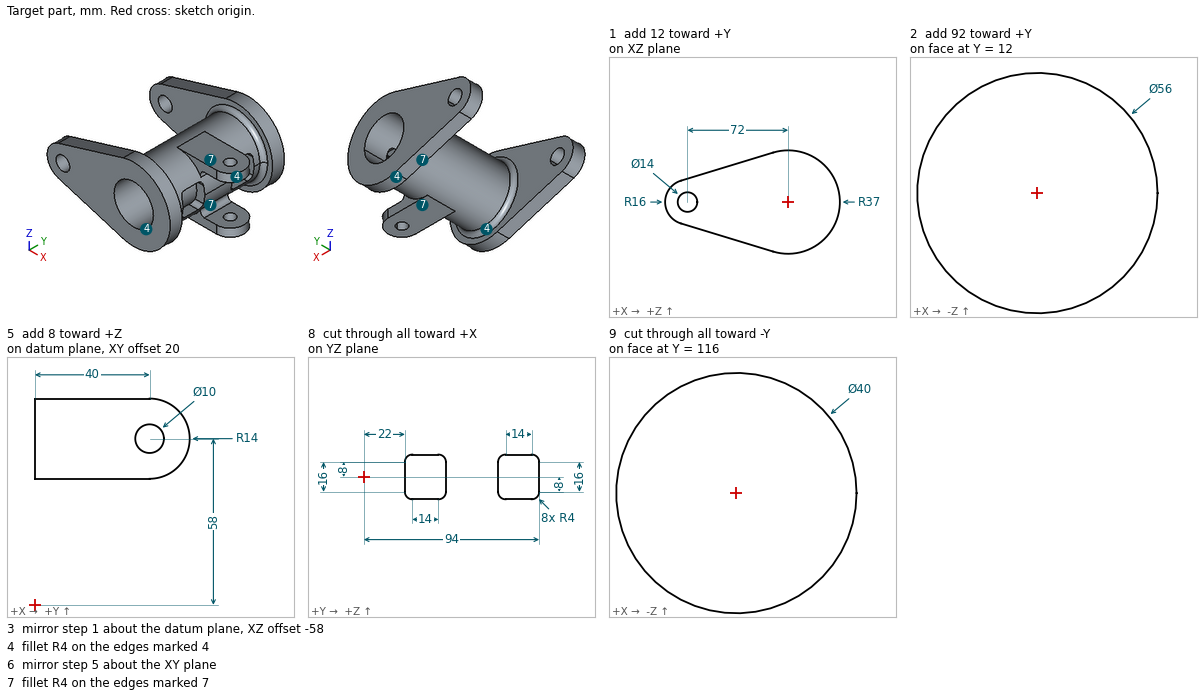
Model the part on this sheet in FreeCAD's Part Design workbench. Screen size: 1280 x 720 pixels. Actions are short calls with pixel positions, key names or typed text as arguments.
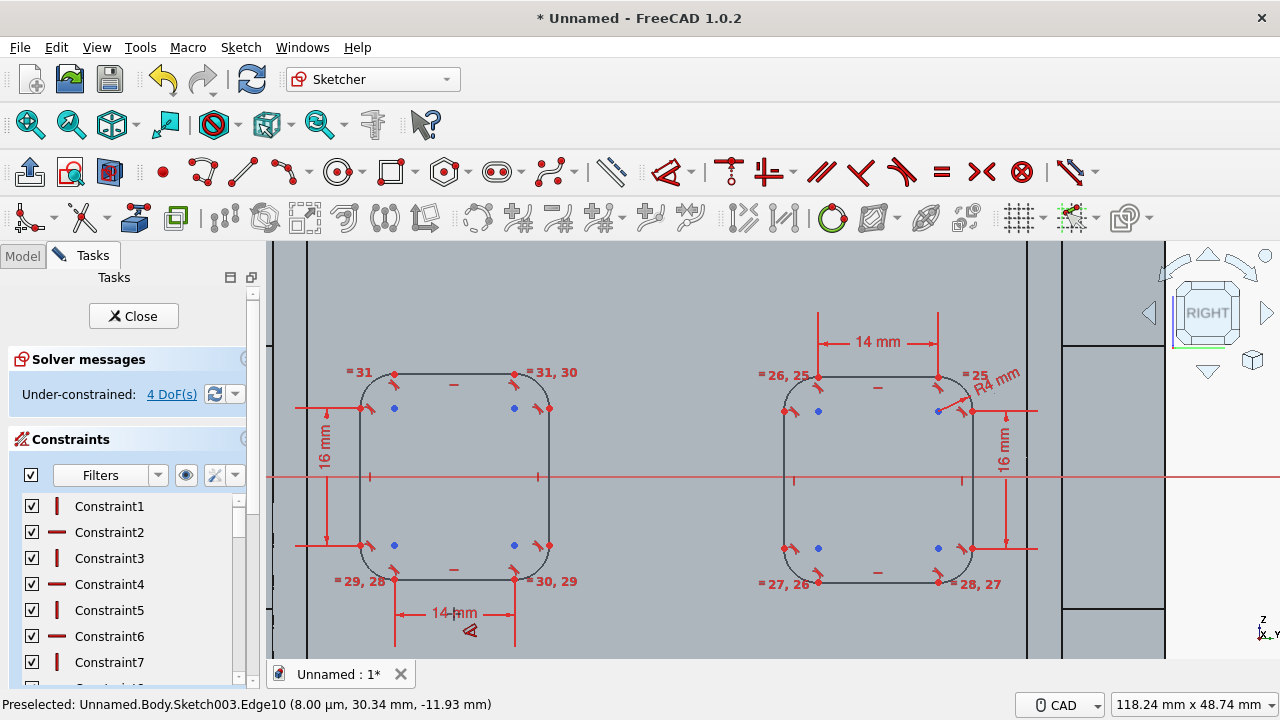
click(973, 549)
click(1007, 513)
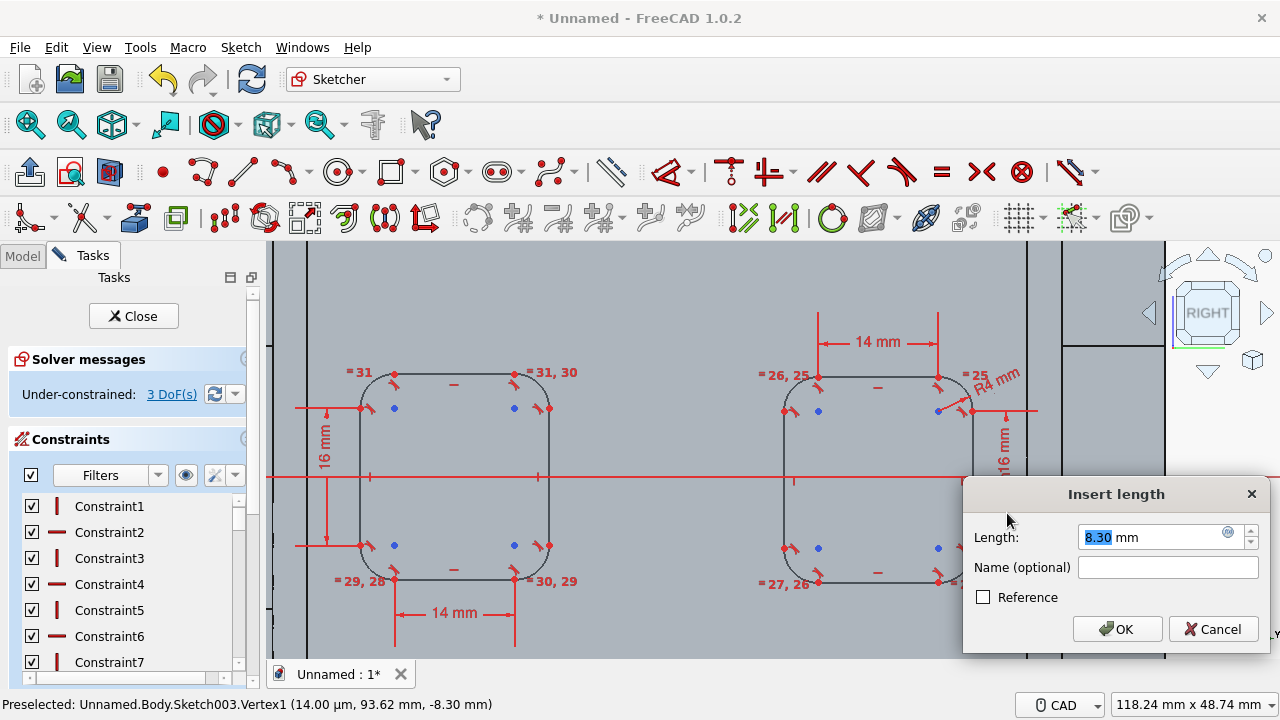
text(8)
key(Return)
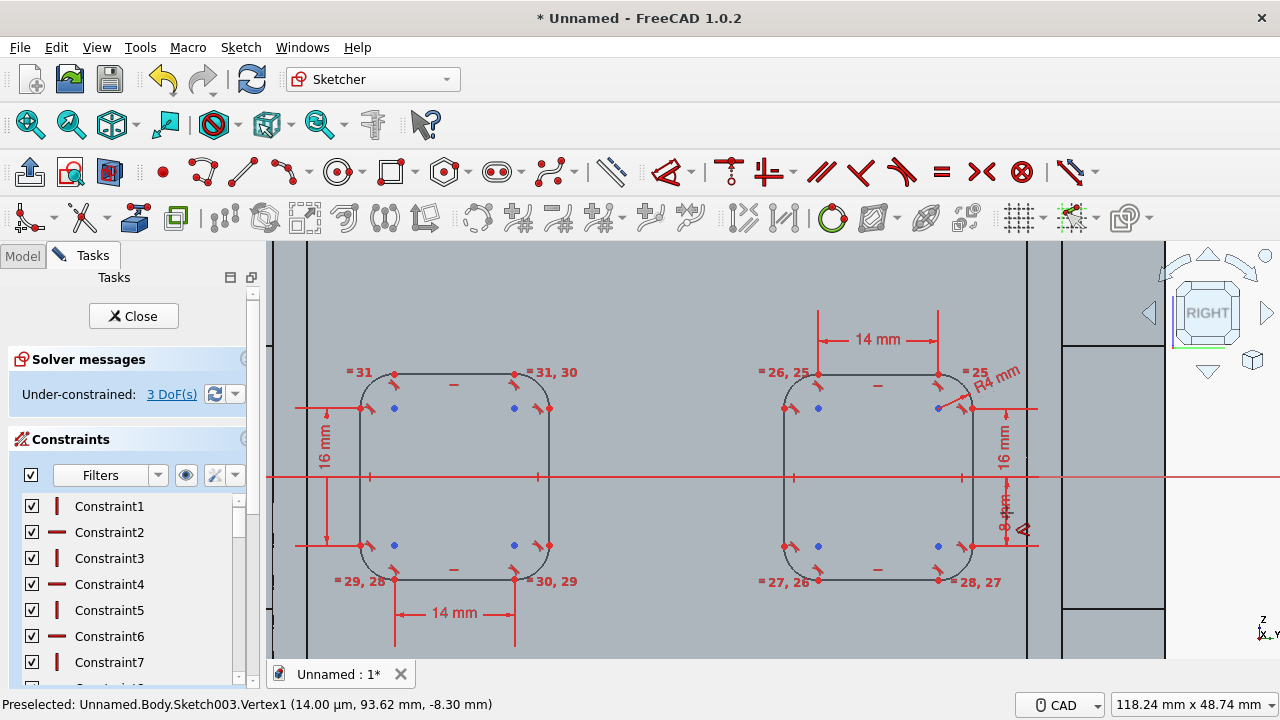
click(360, 408)
click(394, 427)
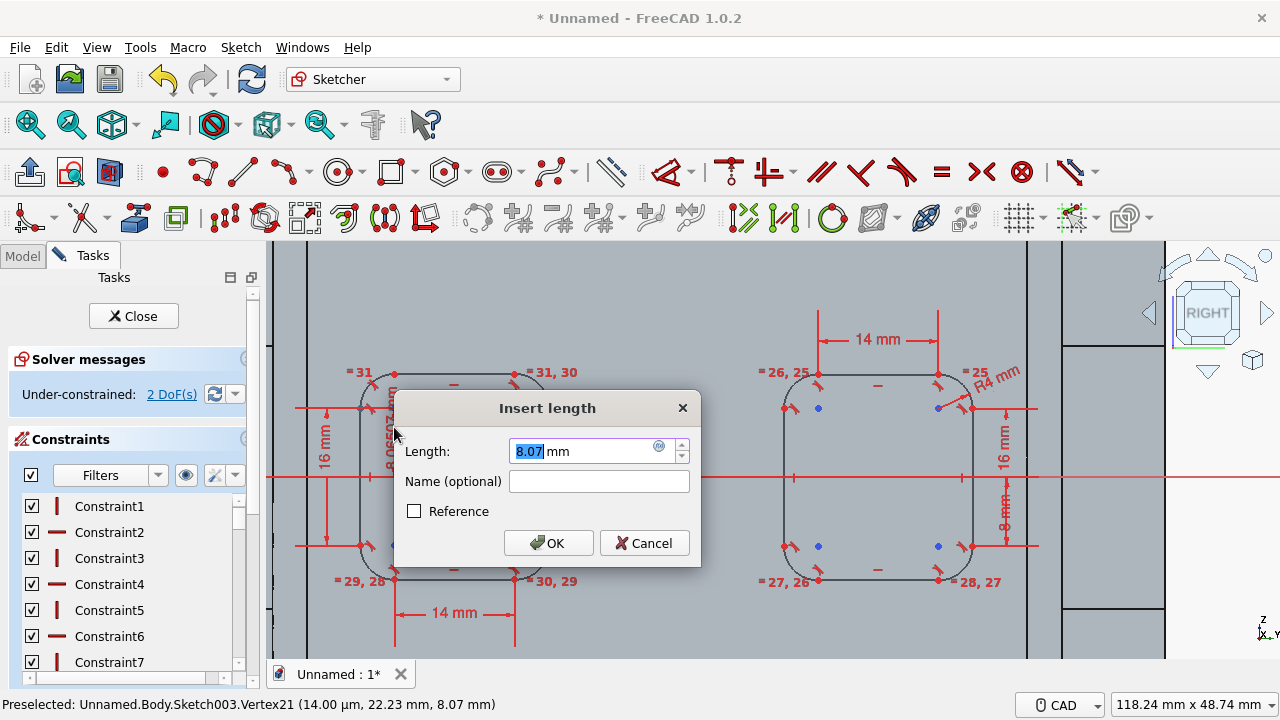
text(8)
key(Return)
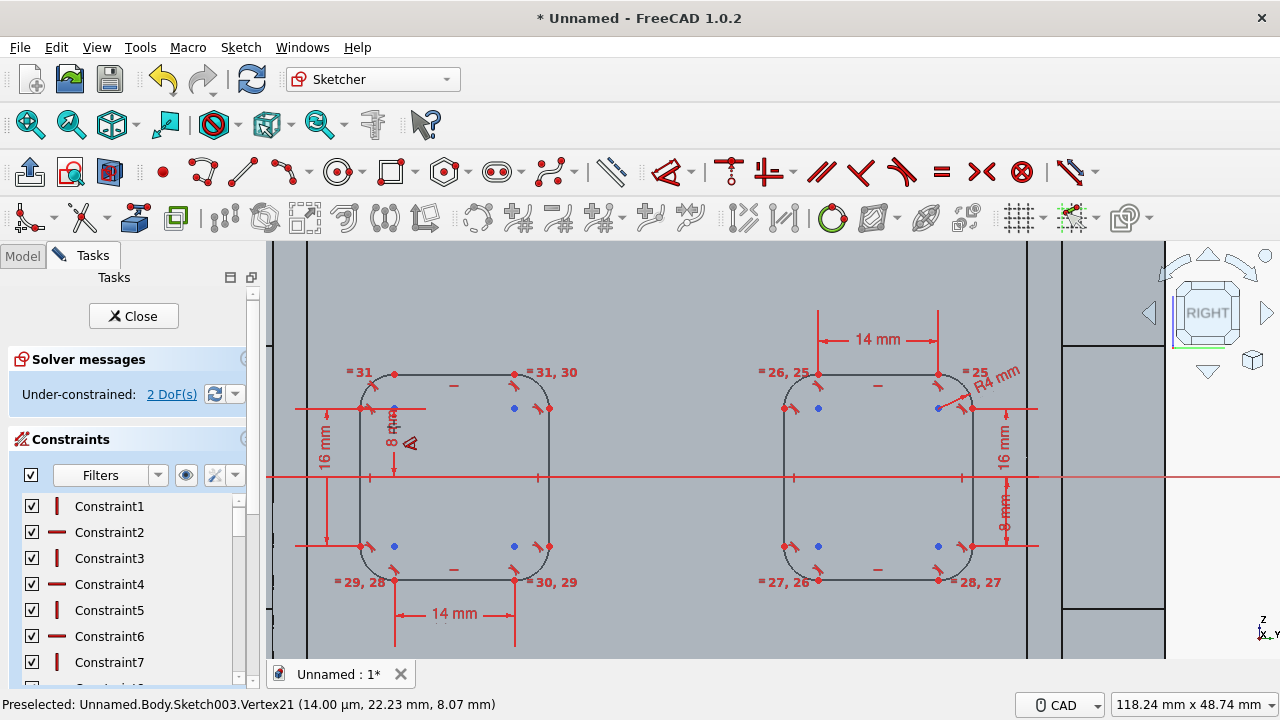
click(973, 546)
click(633, 580)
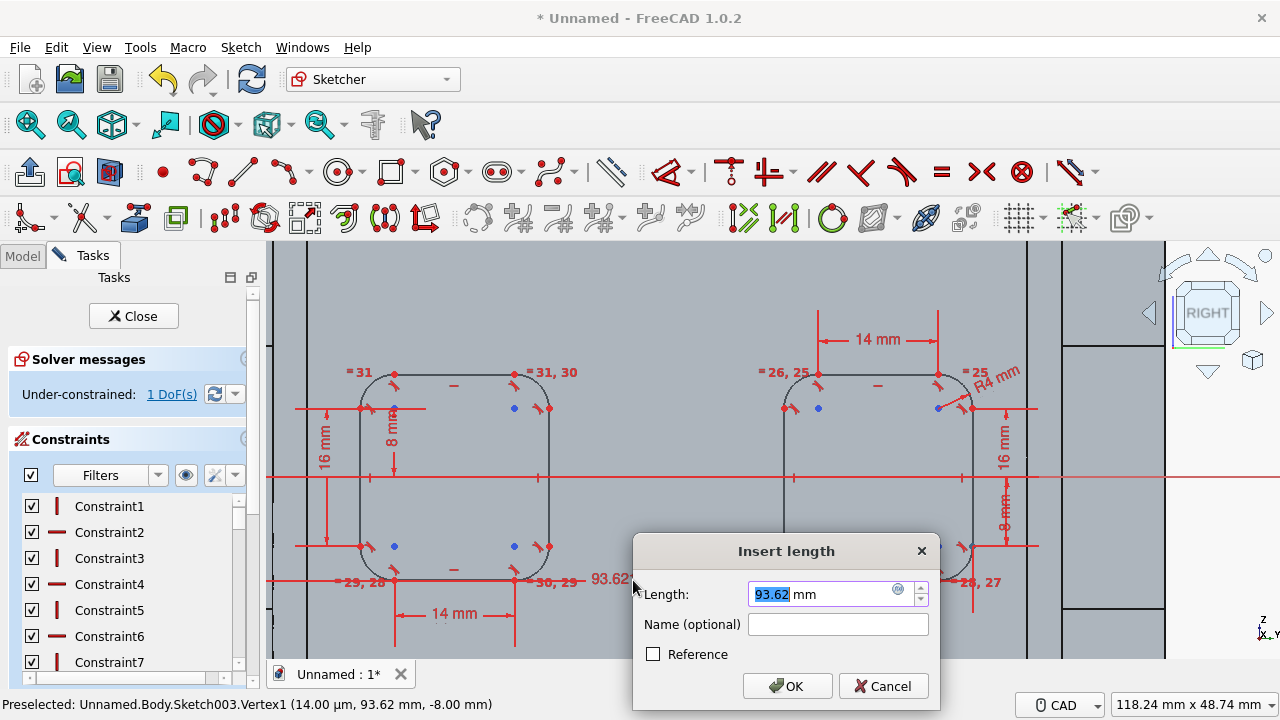
text(94)
key(Return)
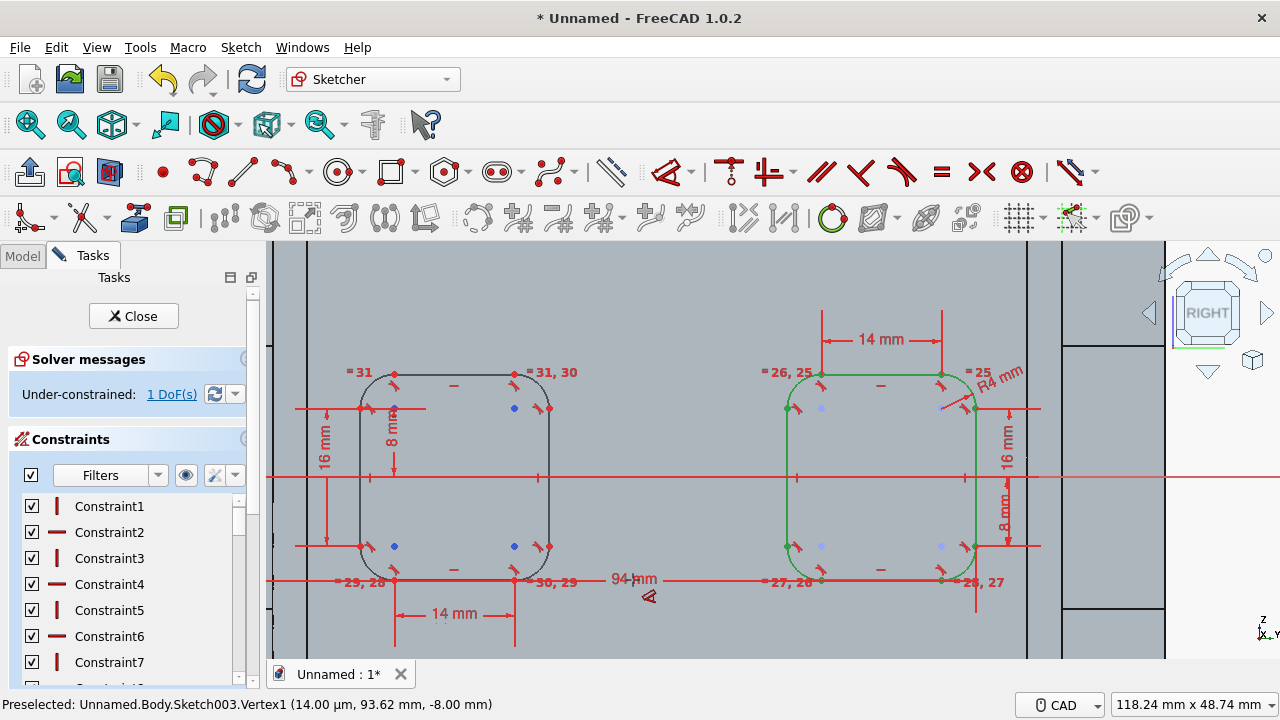
click(360, 409)
click(327, 375)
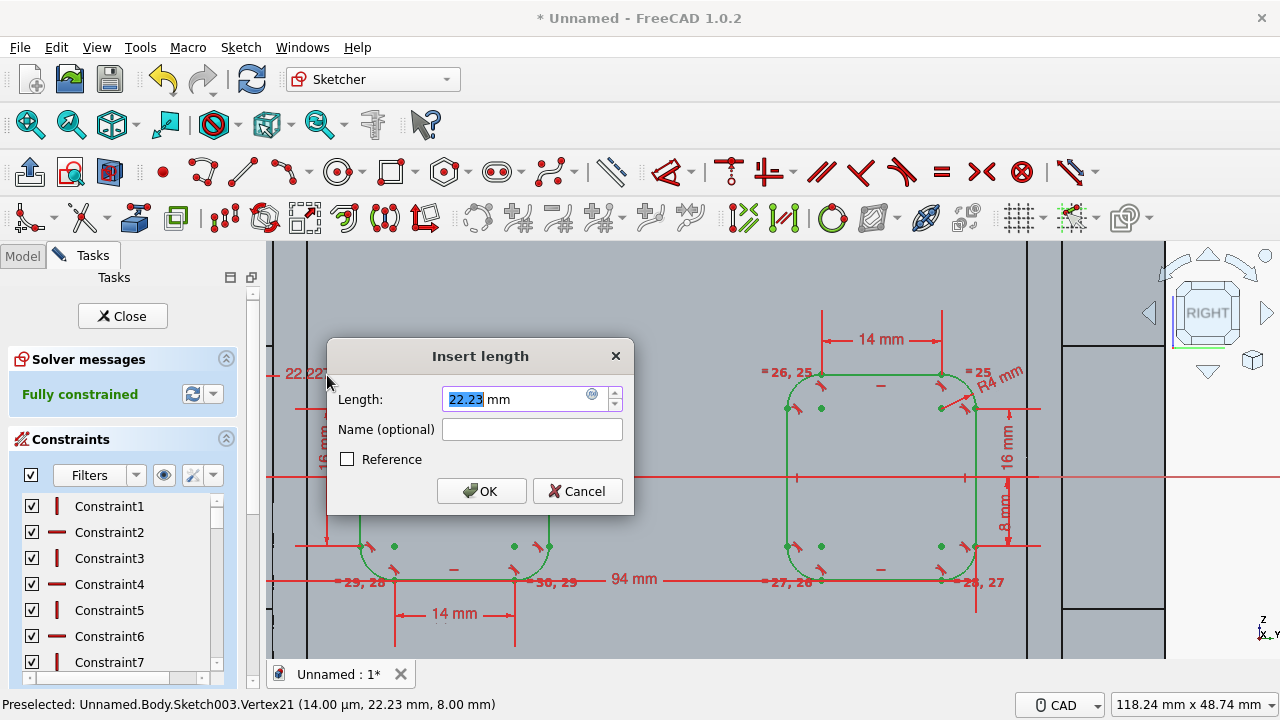
text(22)
key(Return)
key(Escape)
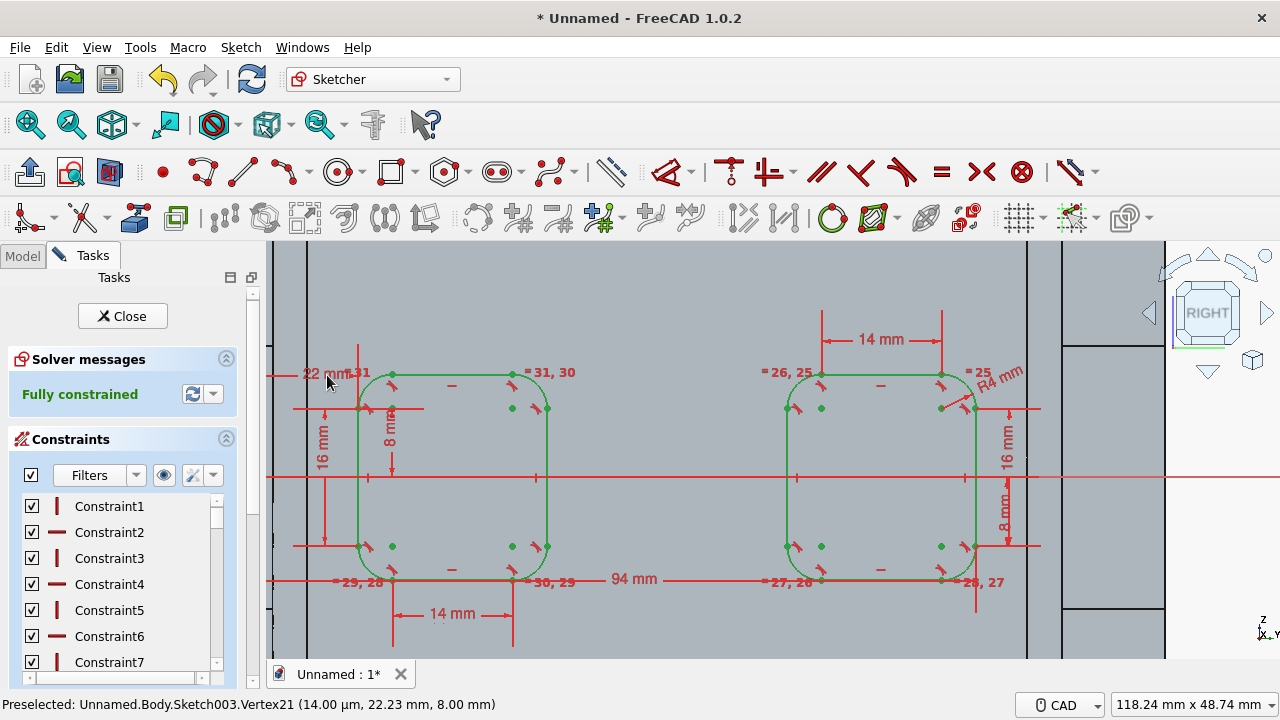
click(123, 316)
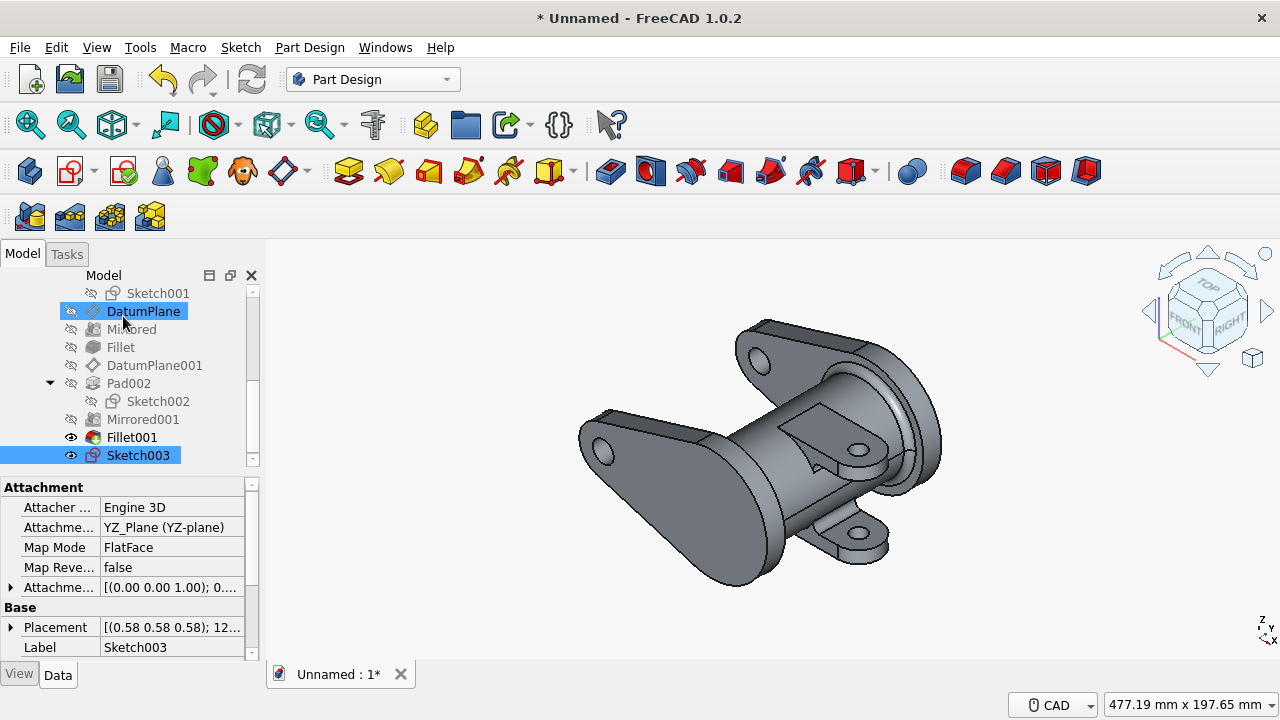
click(612, 172)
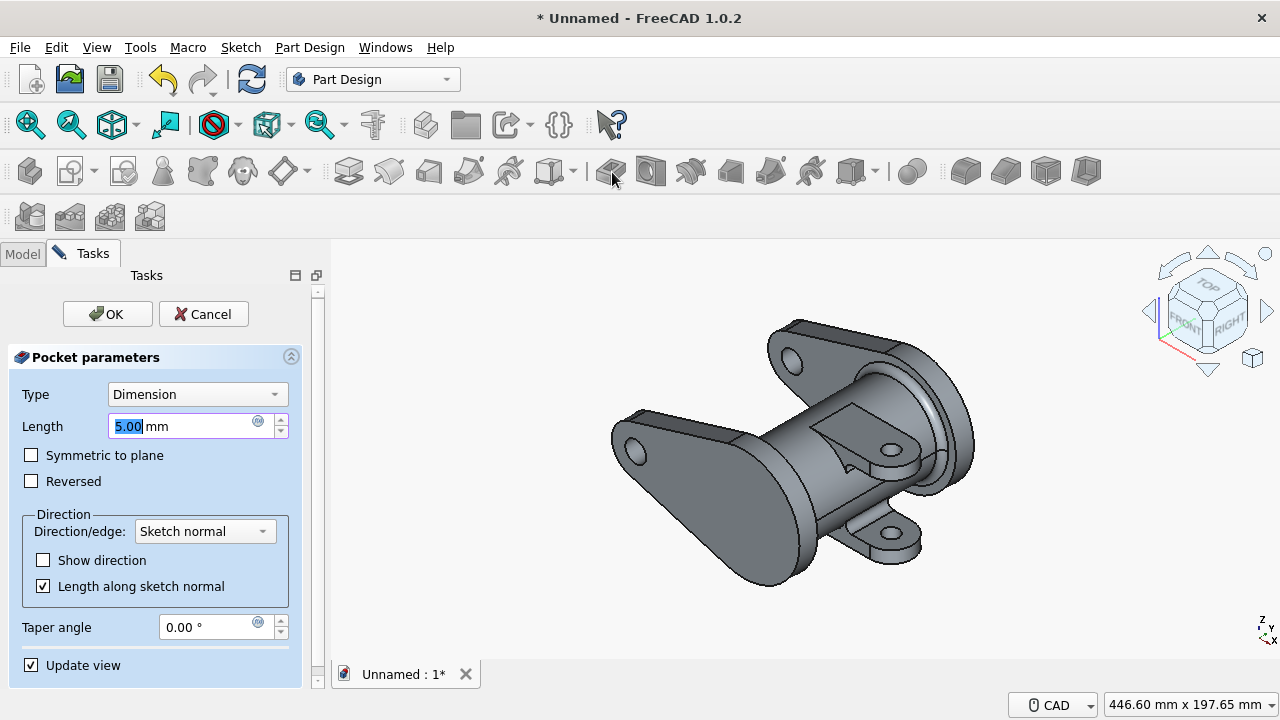
click(198, 394)